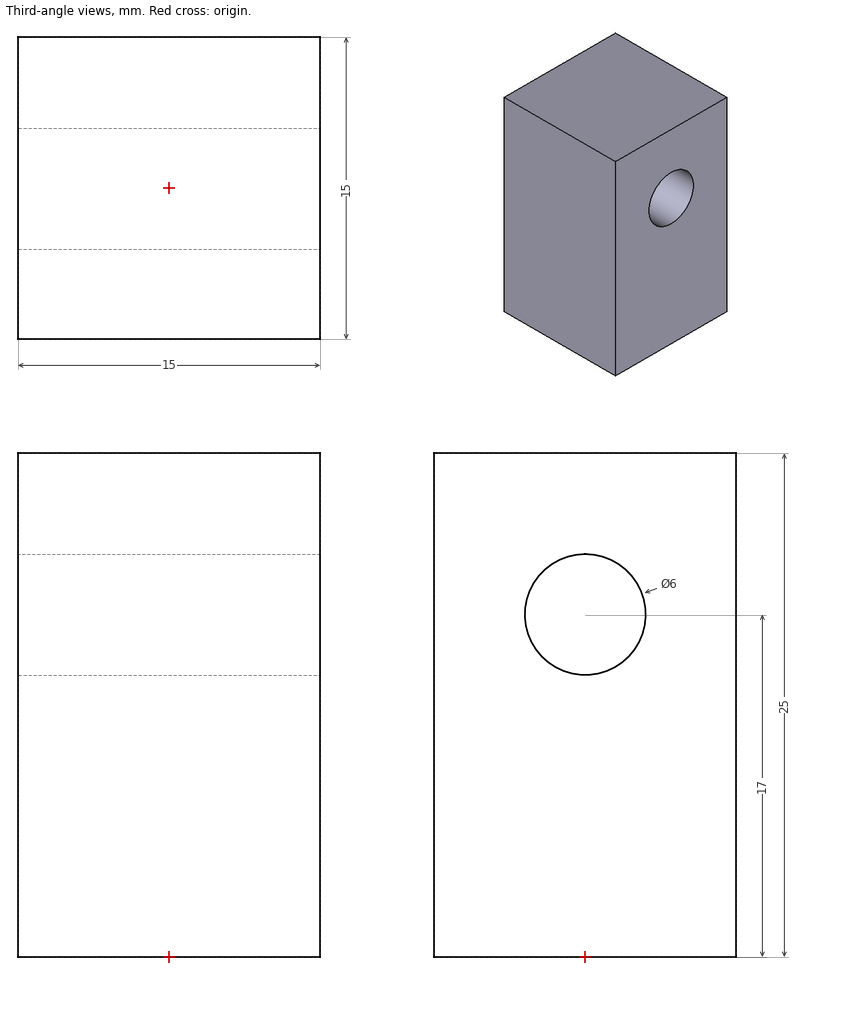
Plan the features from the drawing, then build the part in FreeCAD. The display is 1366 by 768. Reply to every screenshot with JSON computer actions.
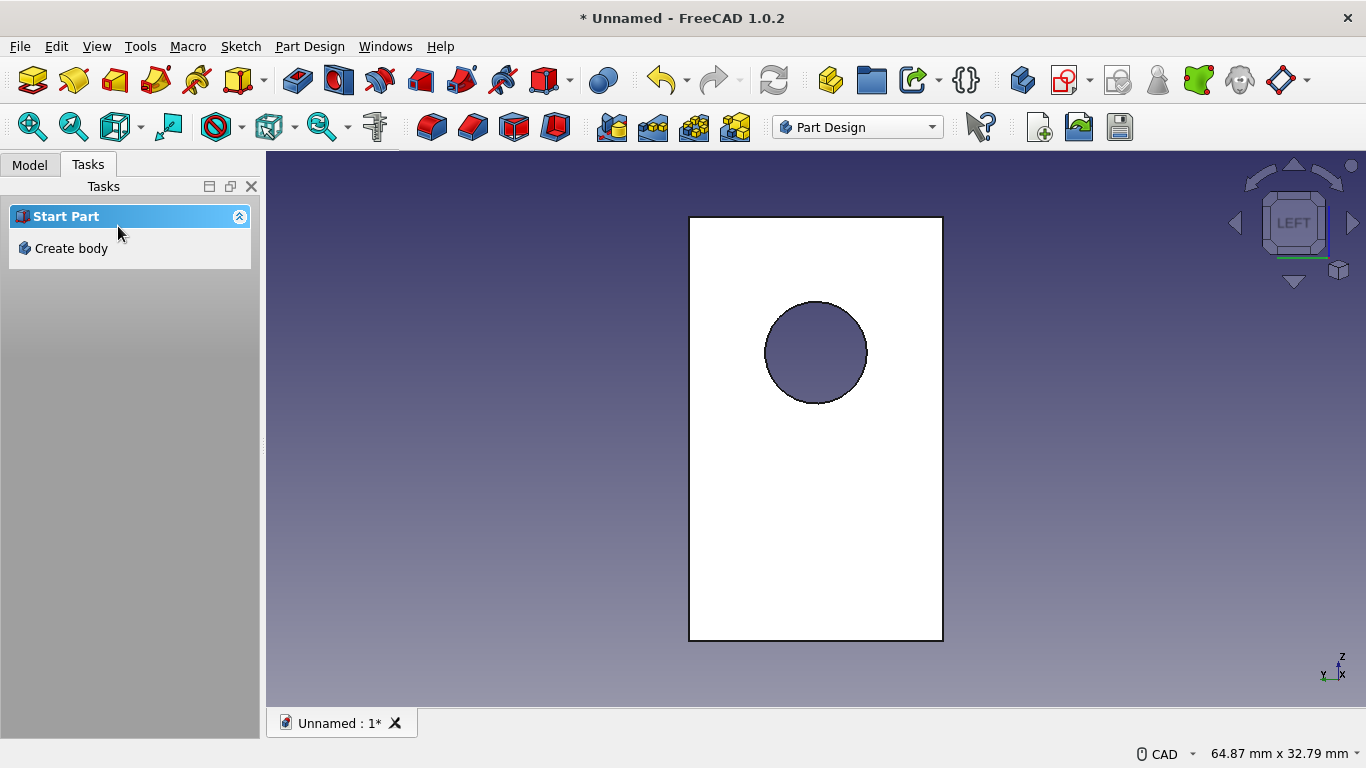
{"action": "key", "text": "0"}